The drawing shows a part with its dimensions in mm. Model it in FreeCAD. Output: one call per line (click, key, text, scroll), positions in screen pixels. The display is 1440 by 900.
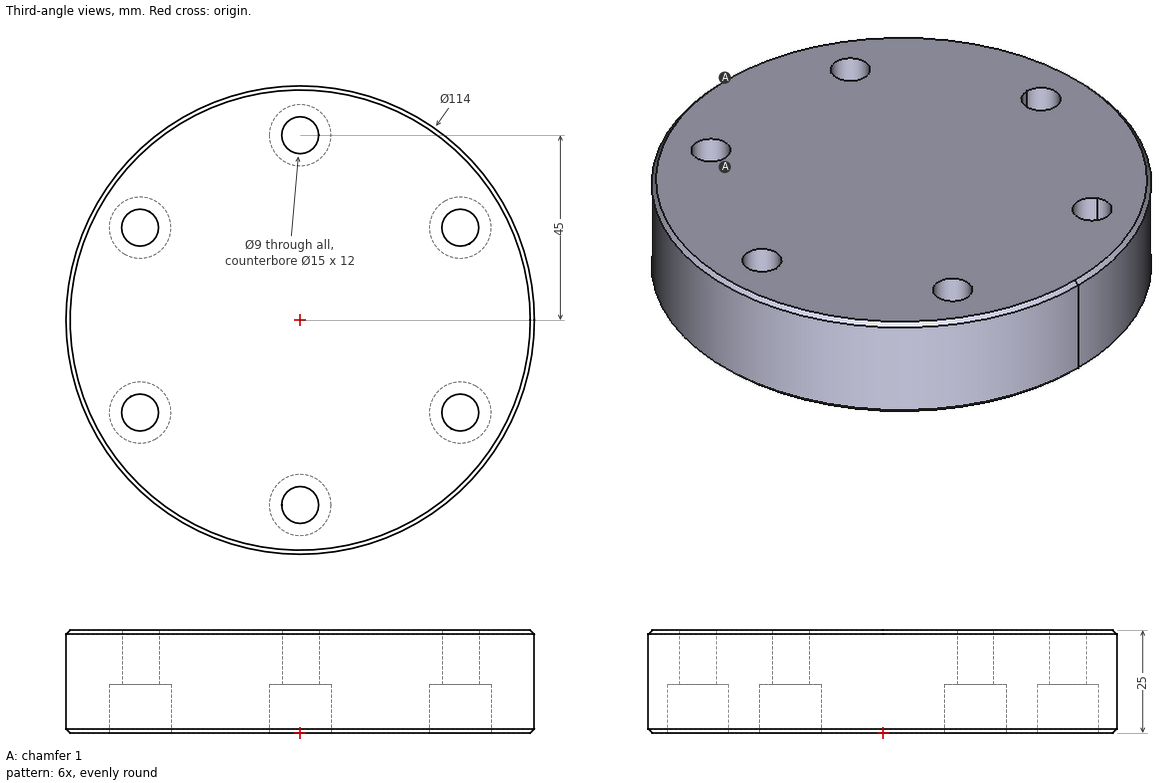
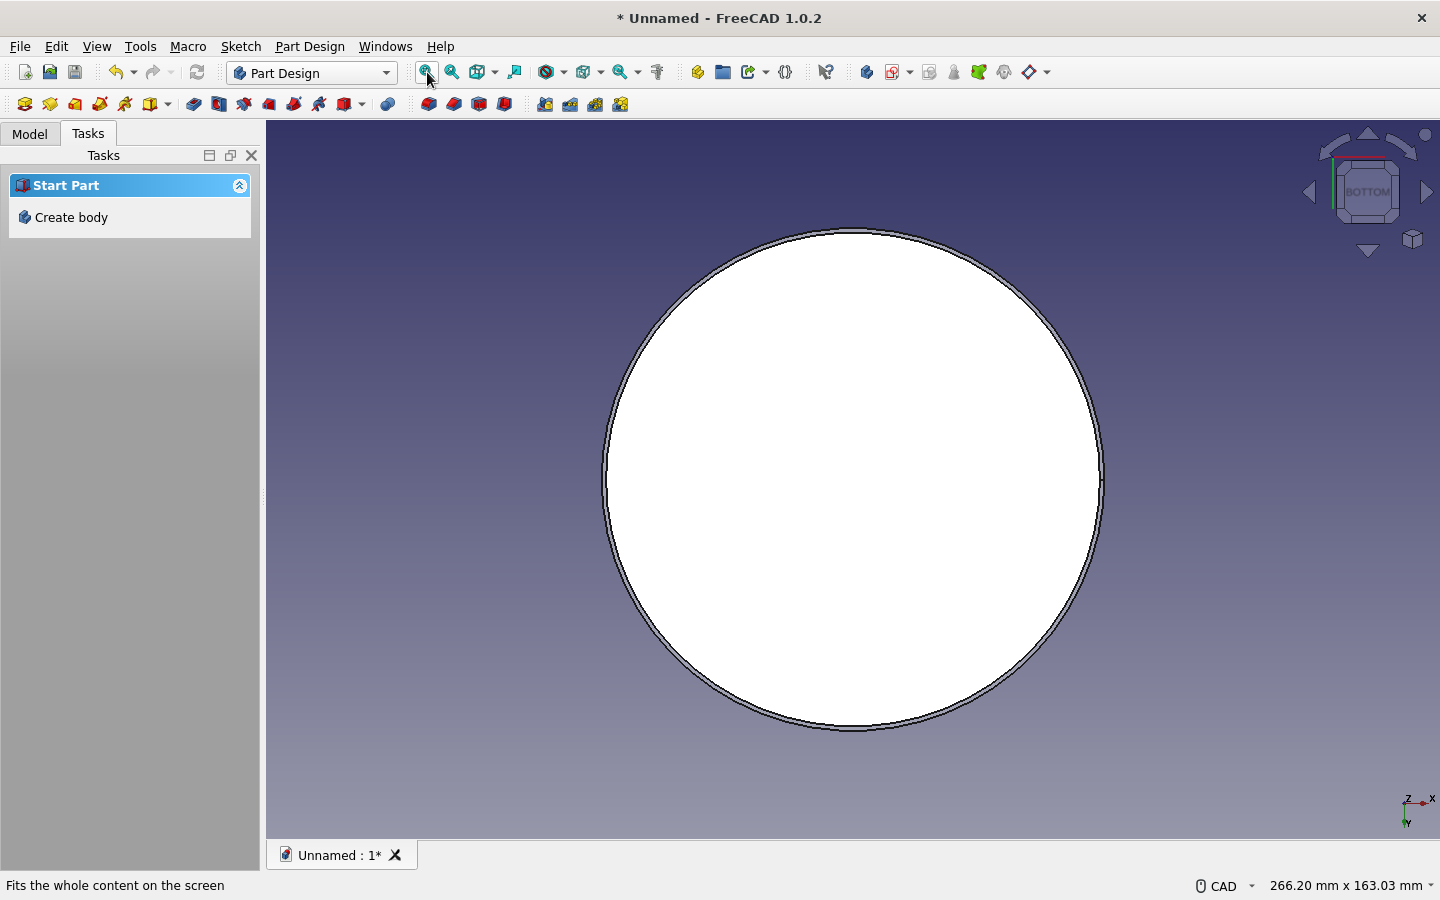
click(853, 478)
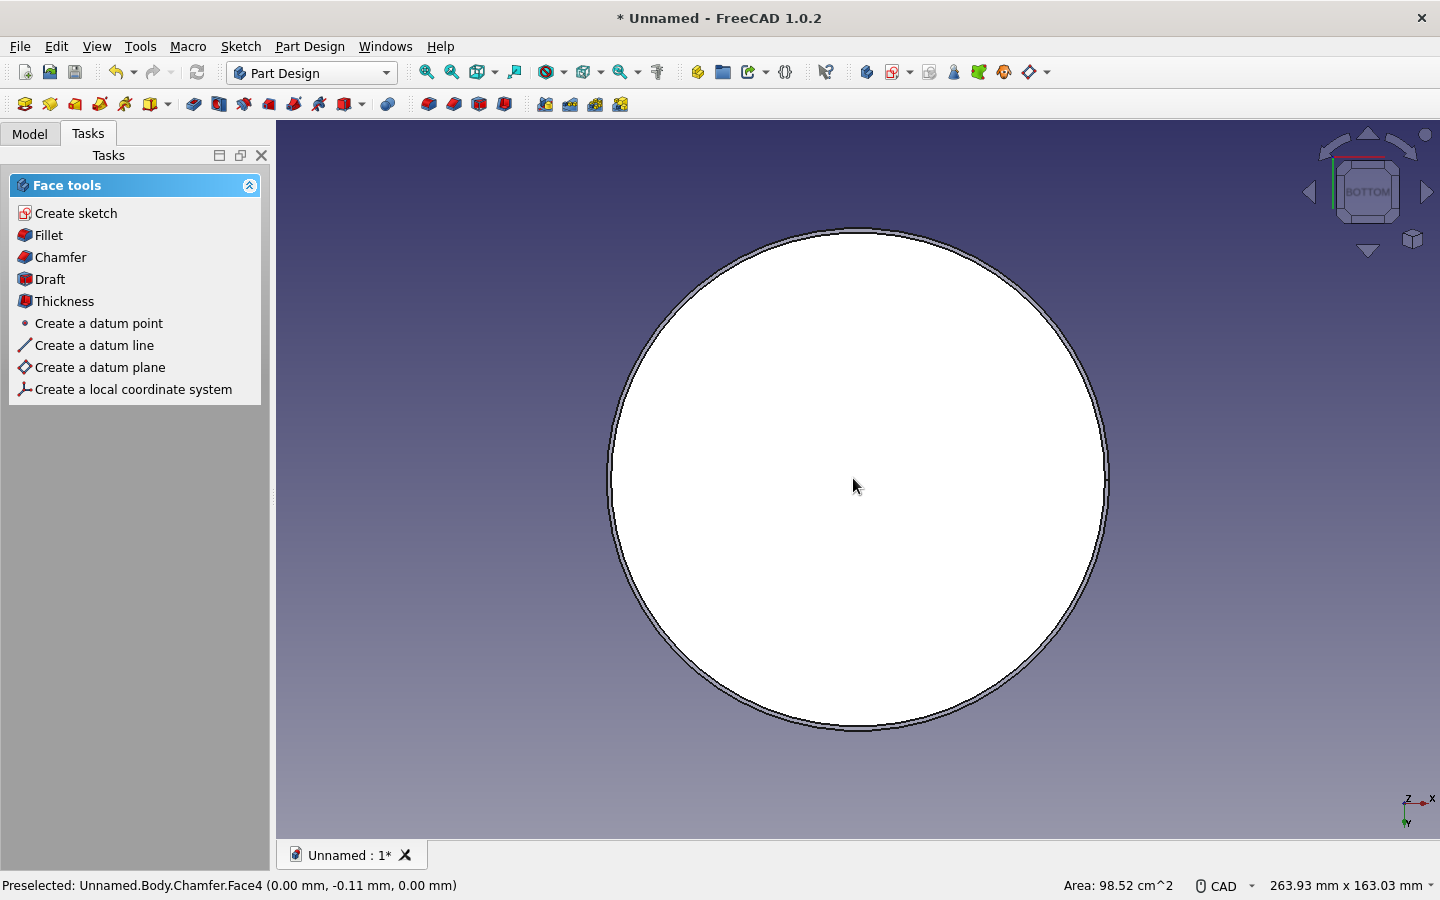
click(892, 72)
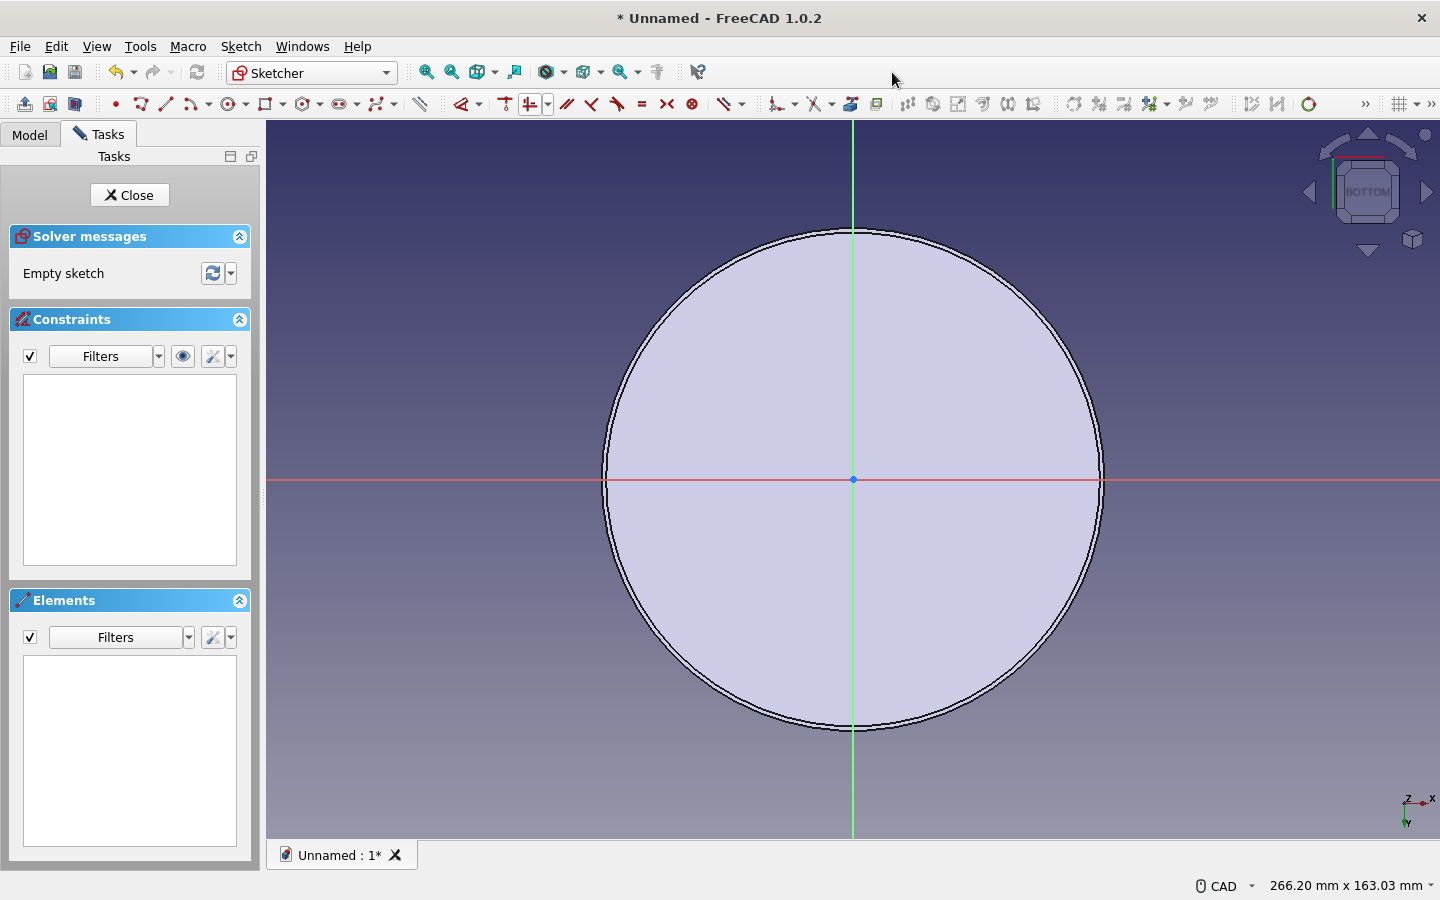
scroll(860, 698, up, 12)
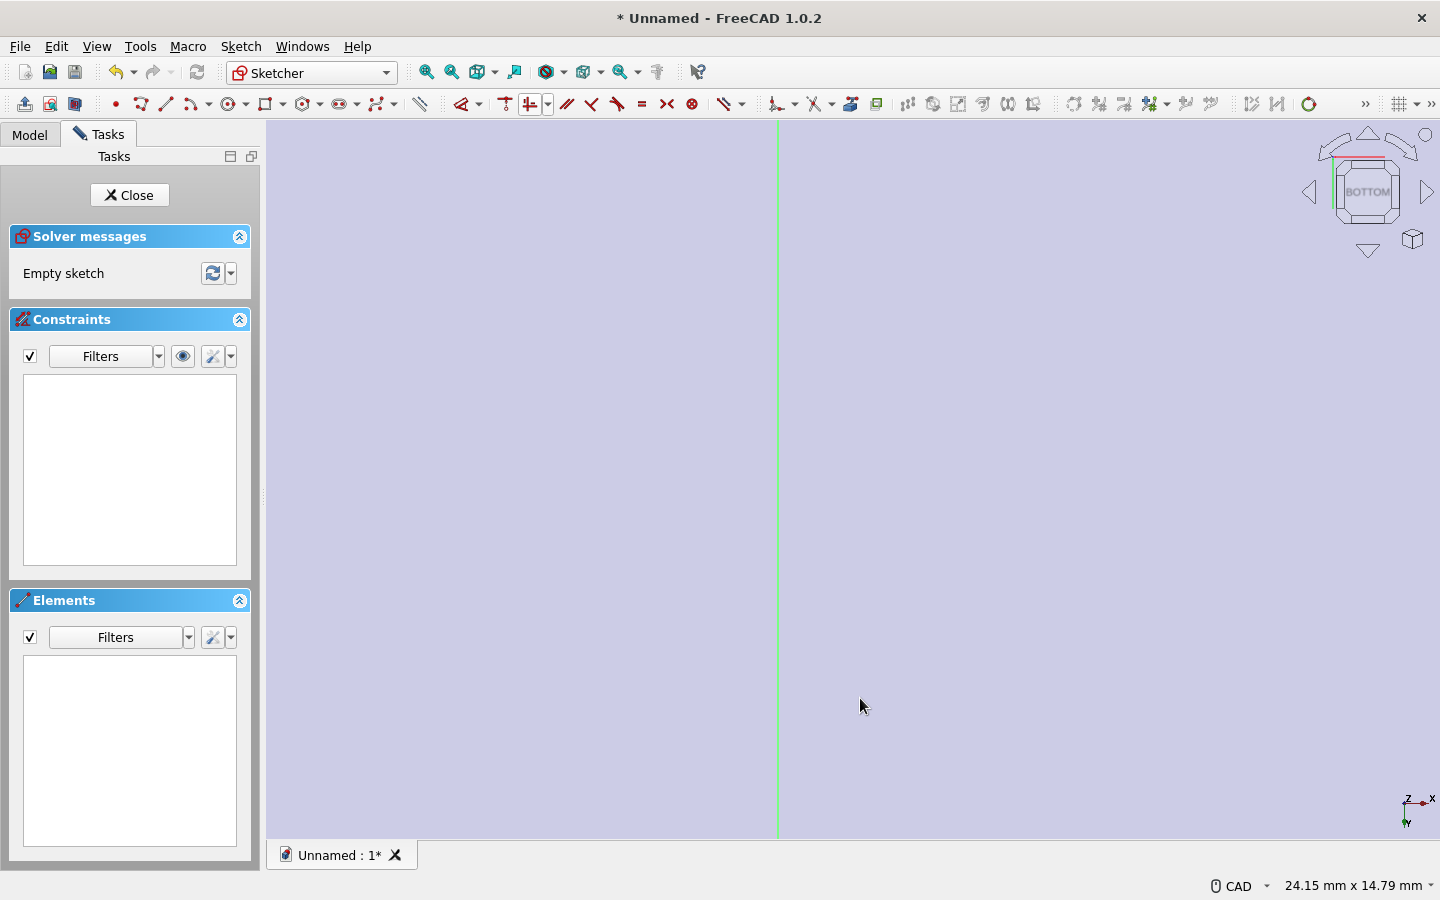
click(228, 104)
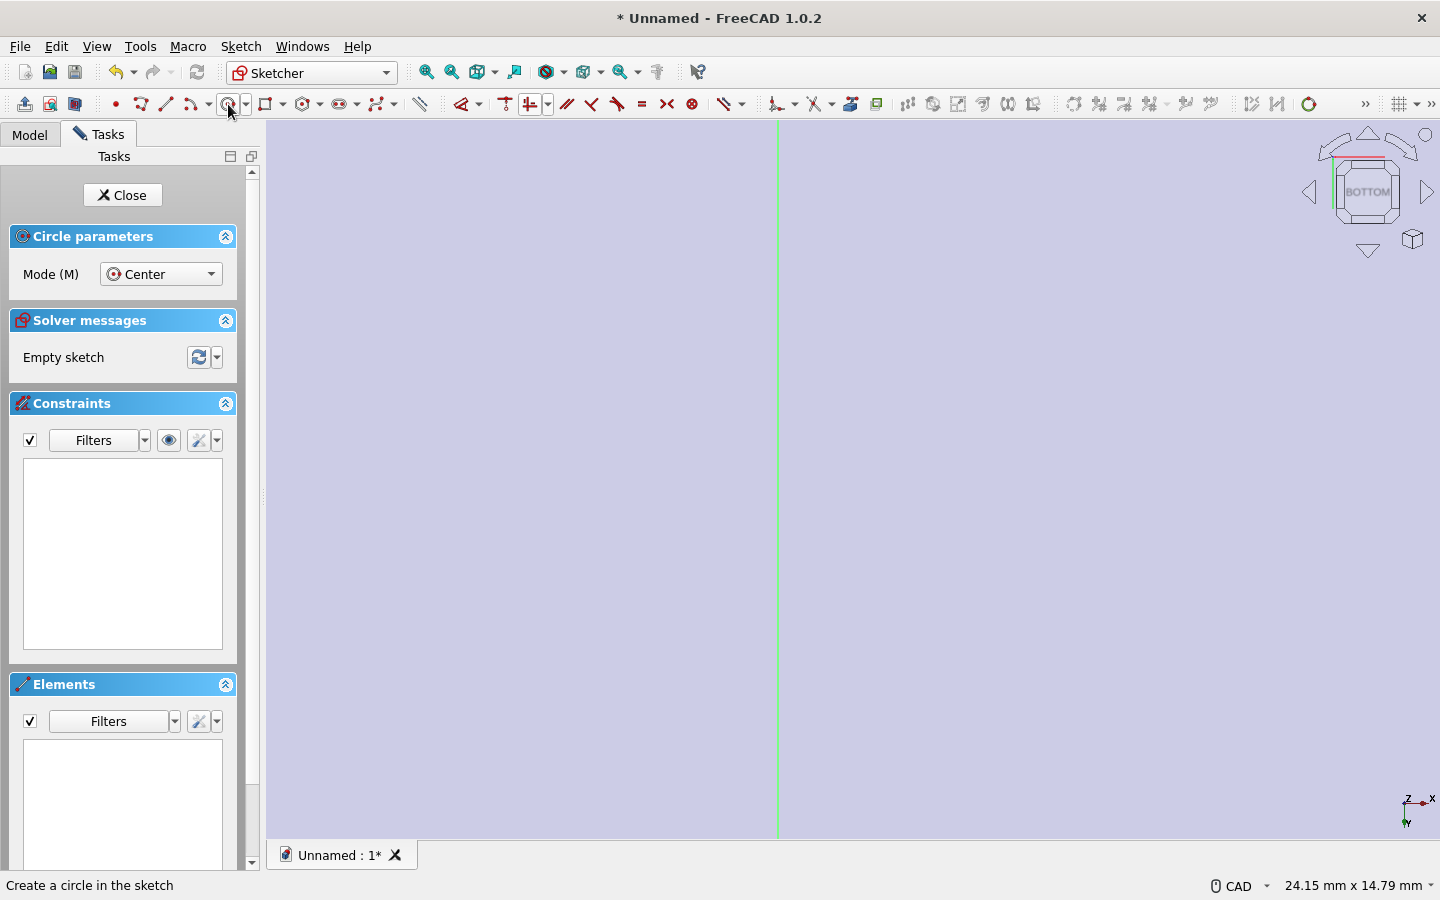
click(778, 469)
move(932, 314)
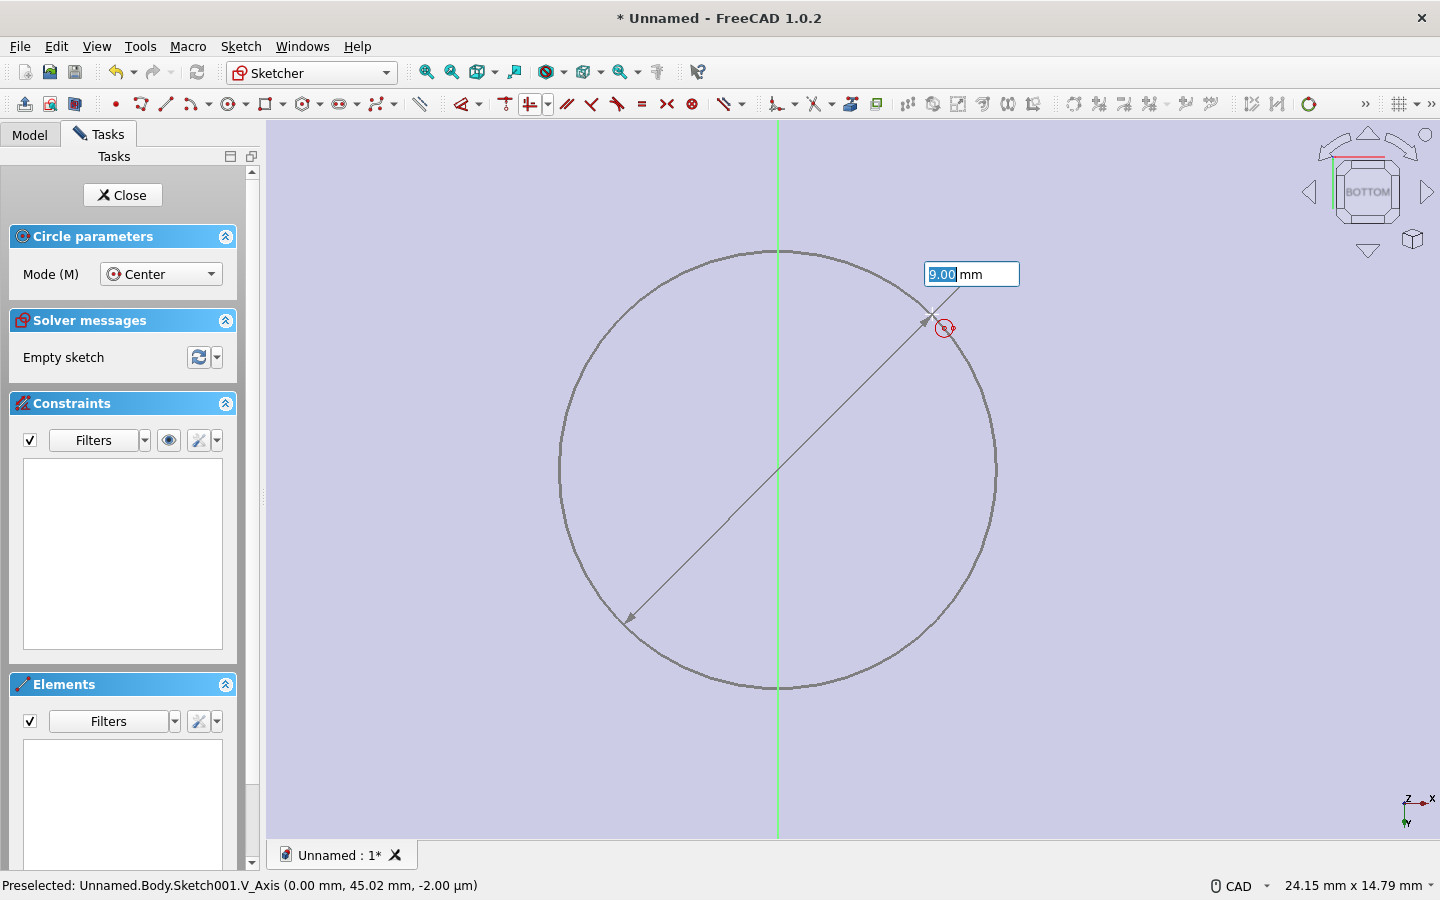
text(9)
key(Return)
key(Escape)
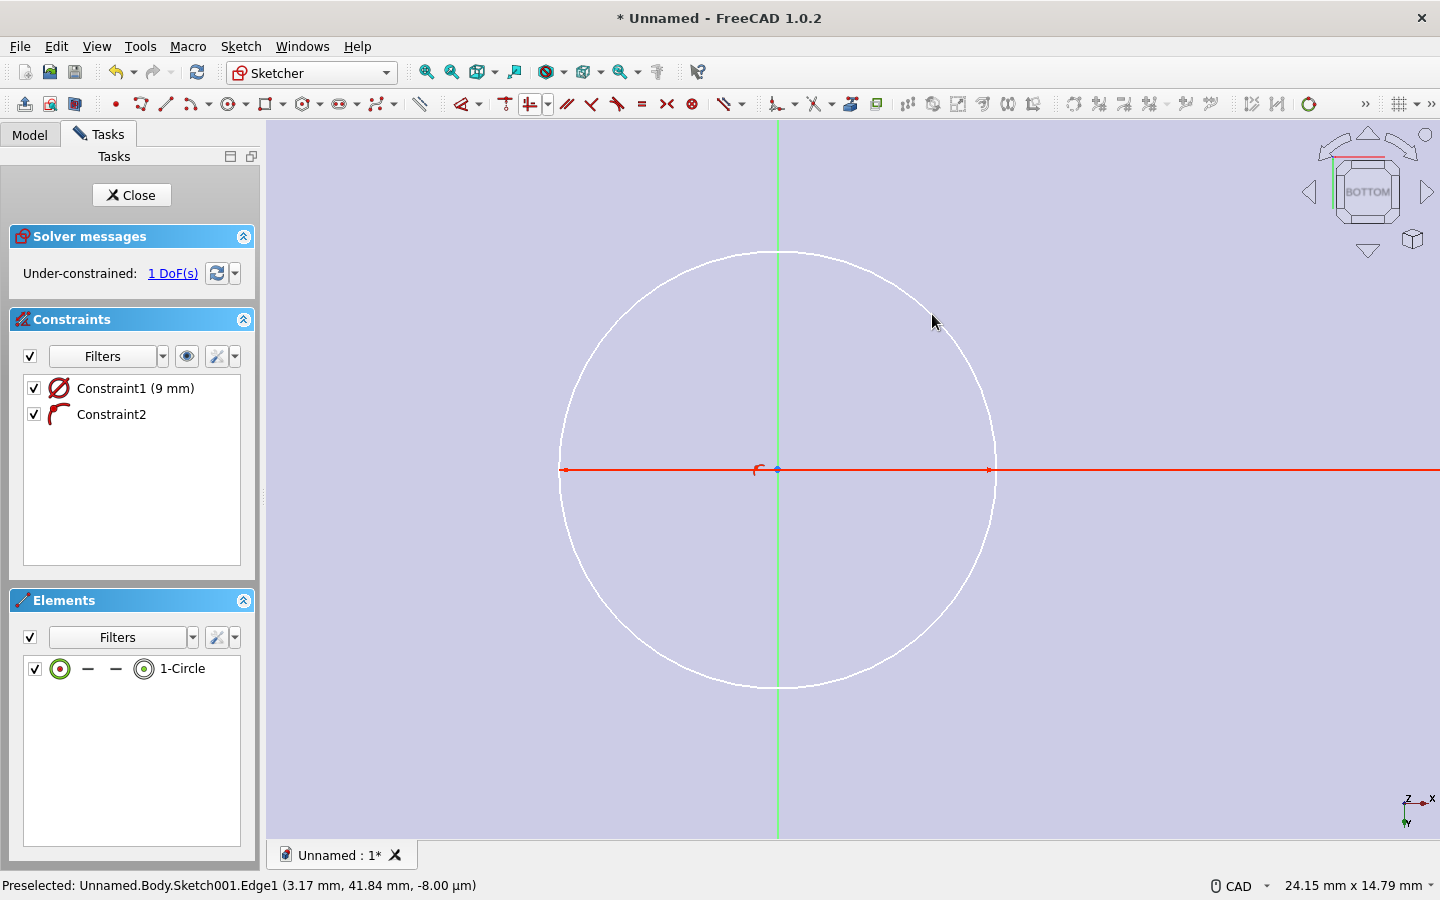
click(460, 104)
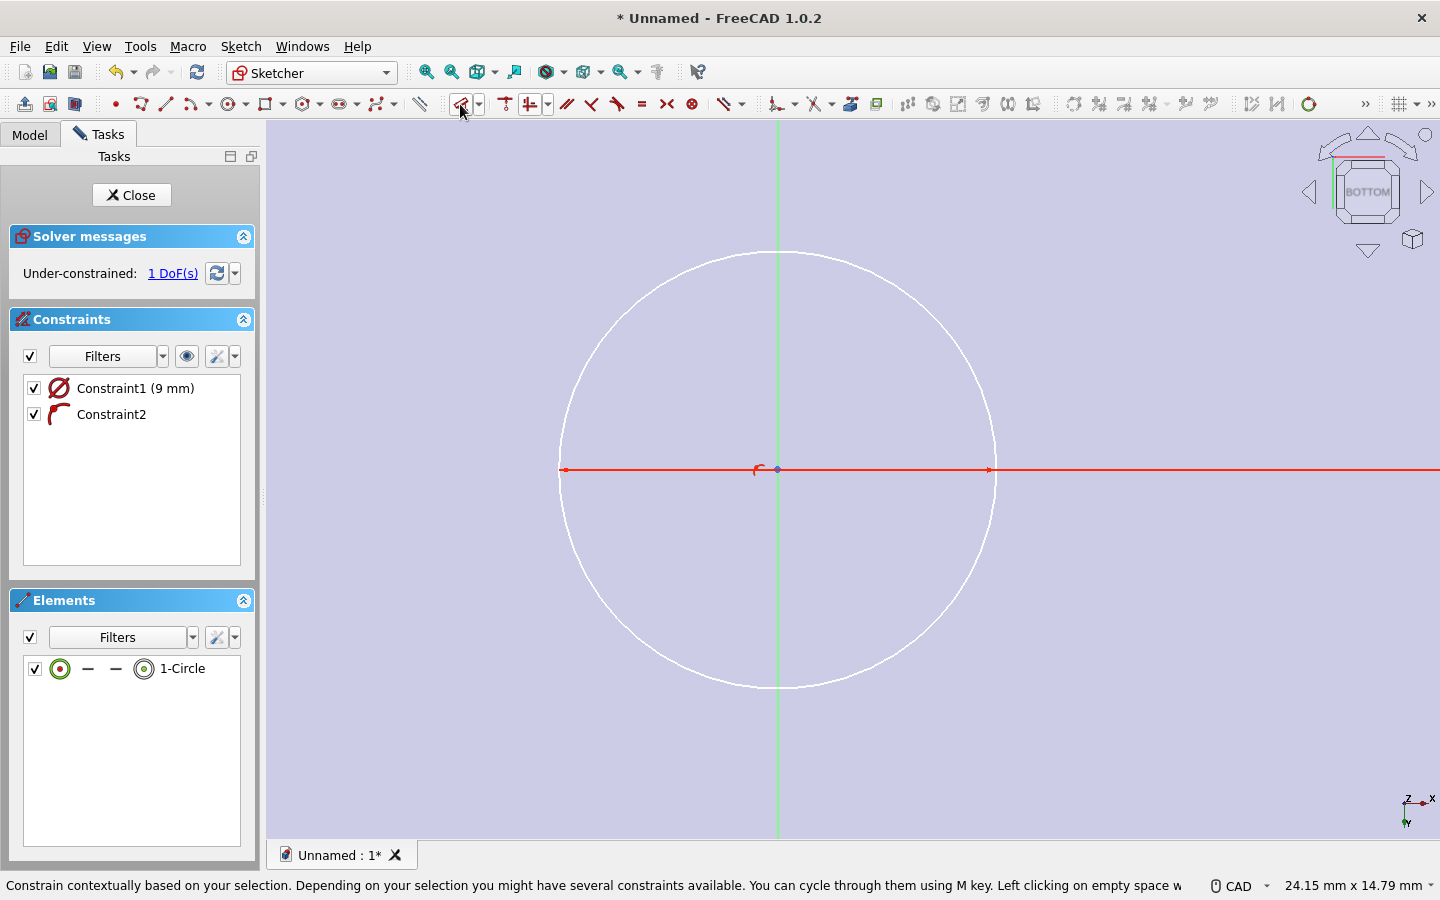
click(778, 470)
click(812, 309)